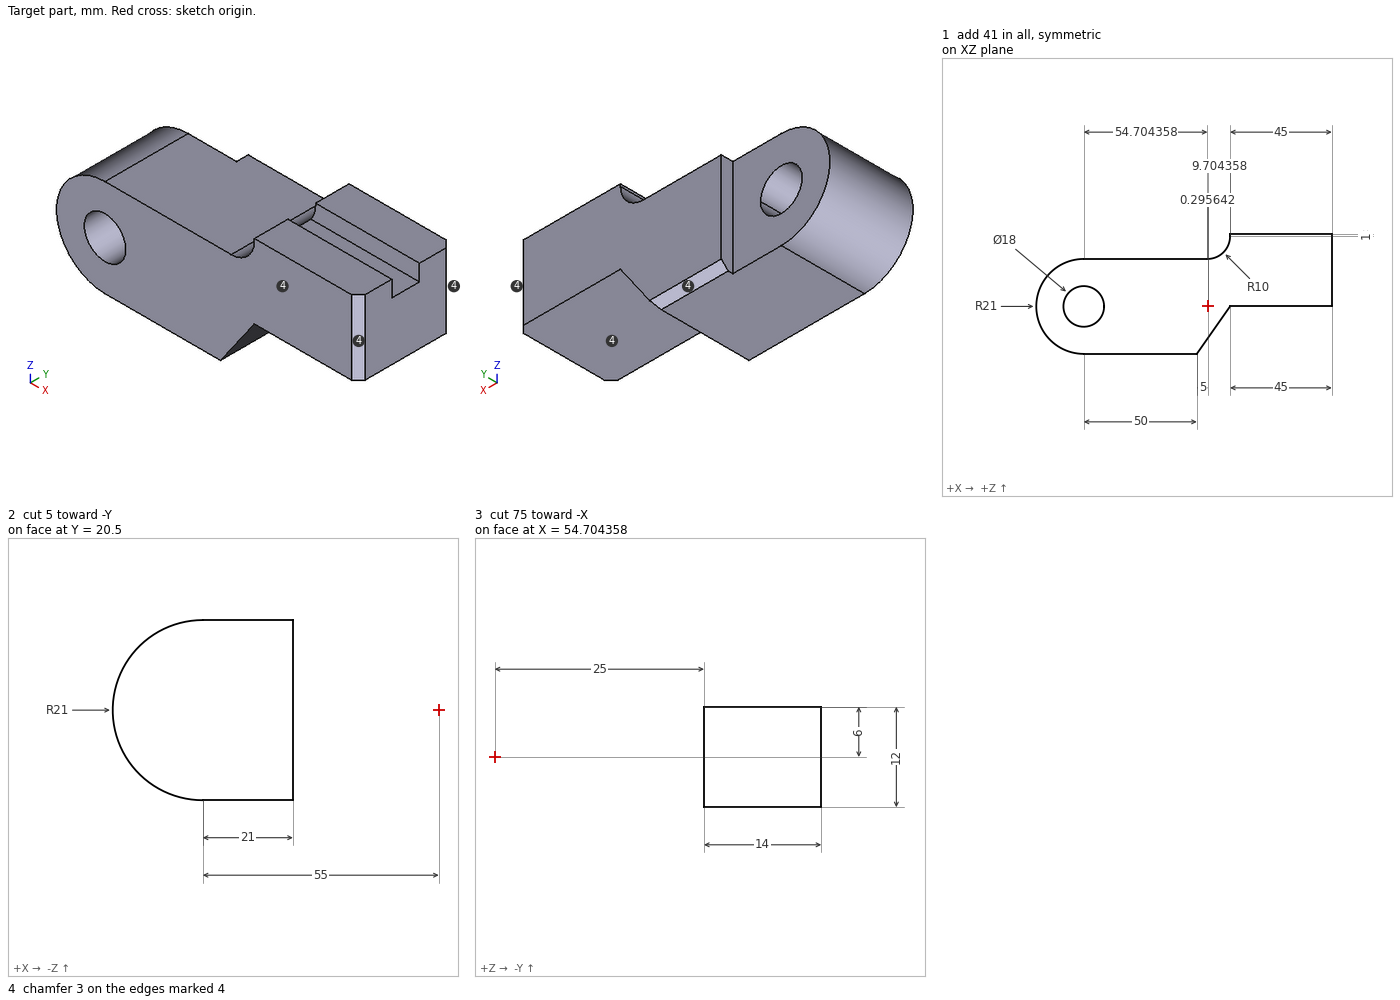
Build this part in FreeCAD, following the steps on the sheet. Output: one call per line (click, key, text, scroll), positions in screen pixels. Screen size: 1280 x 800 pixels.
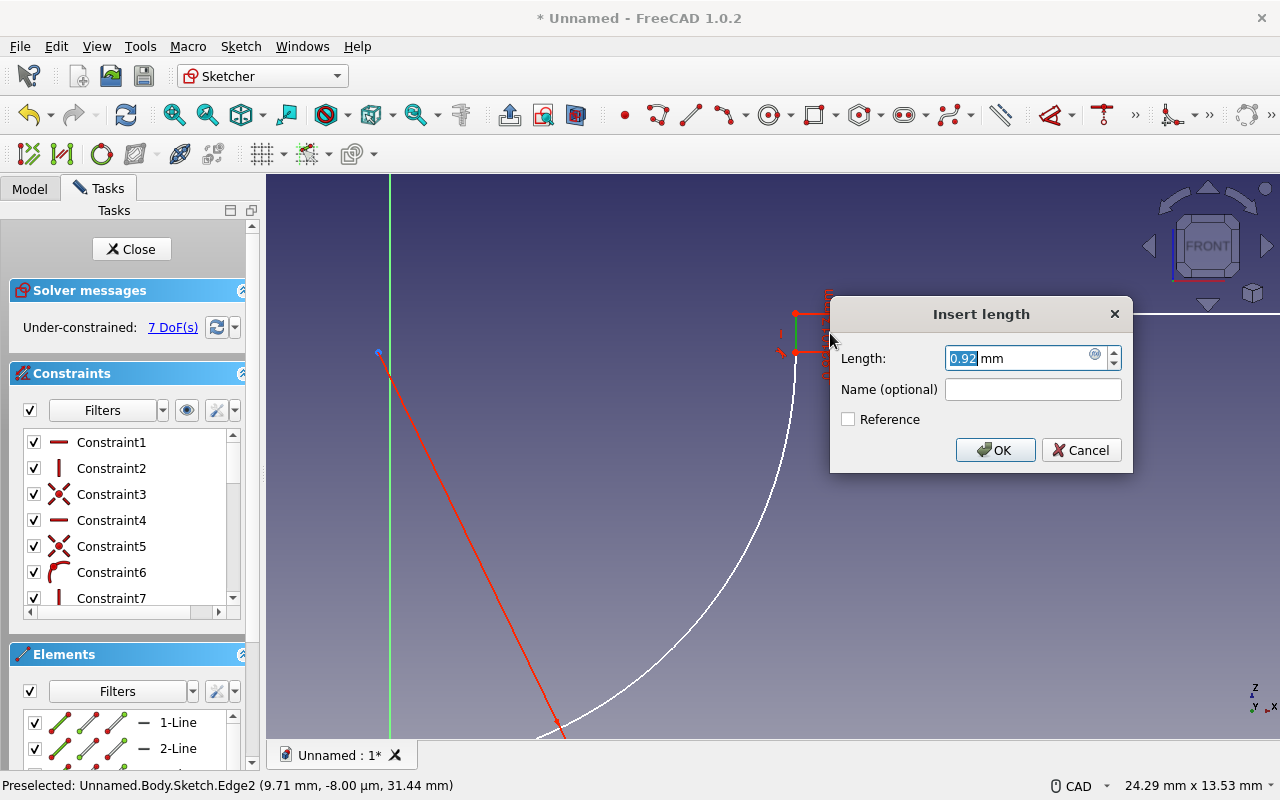
text(1)
key(Return)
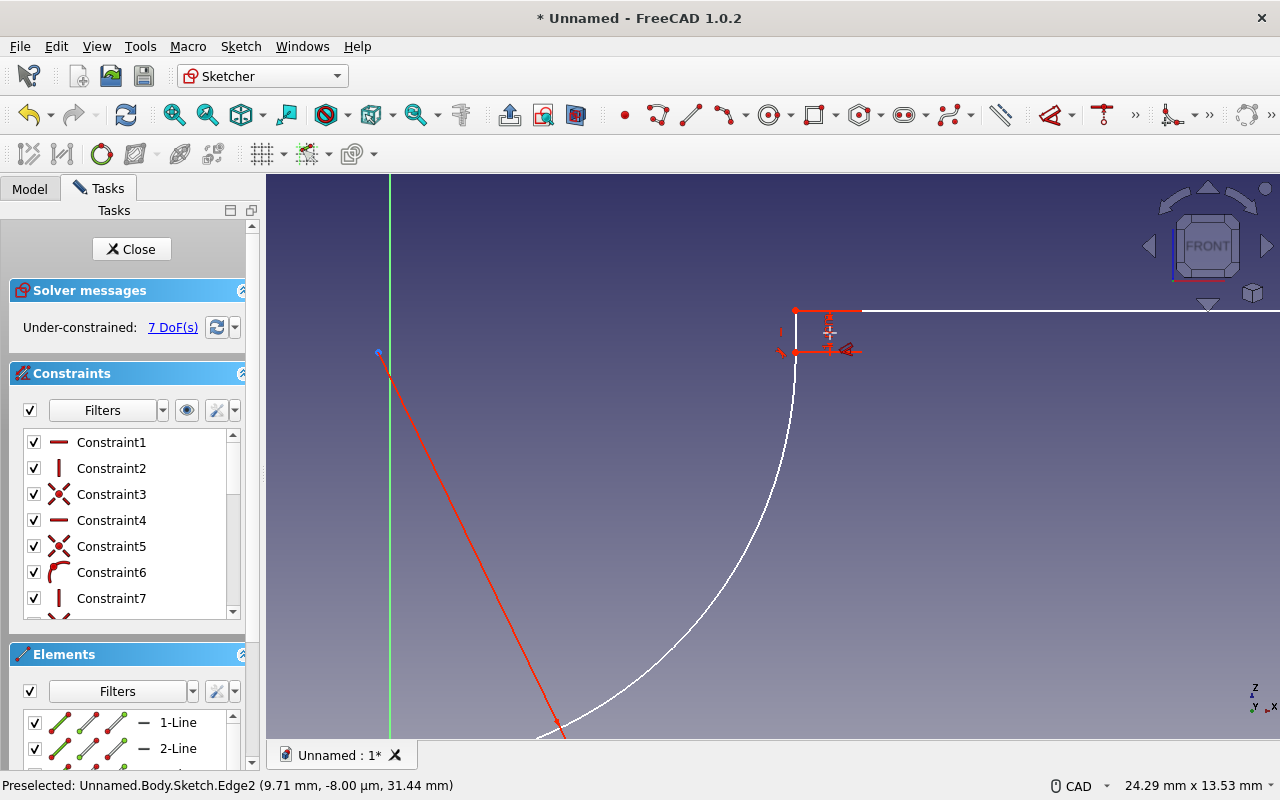
scroll(799, 337, down, 11)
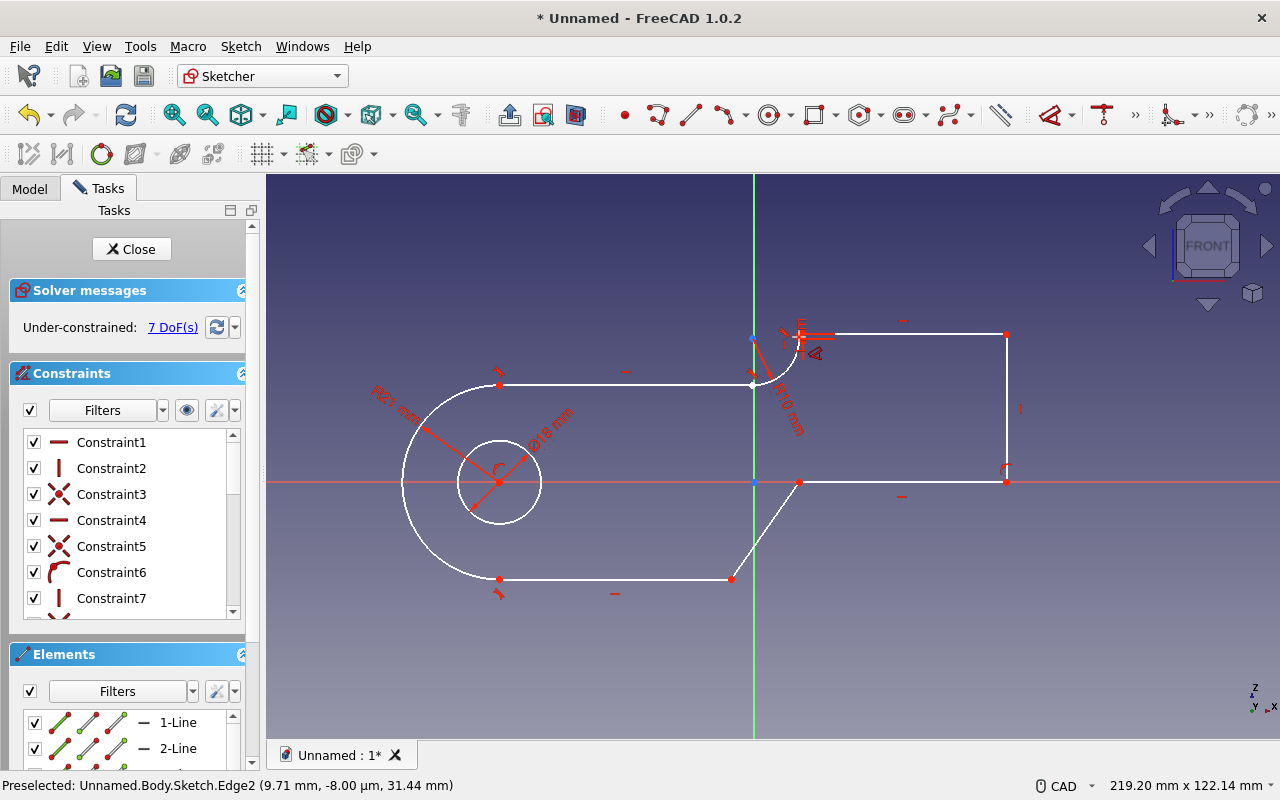
click(861, 334)
click(903, 300)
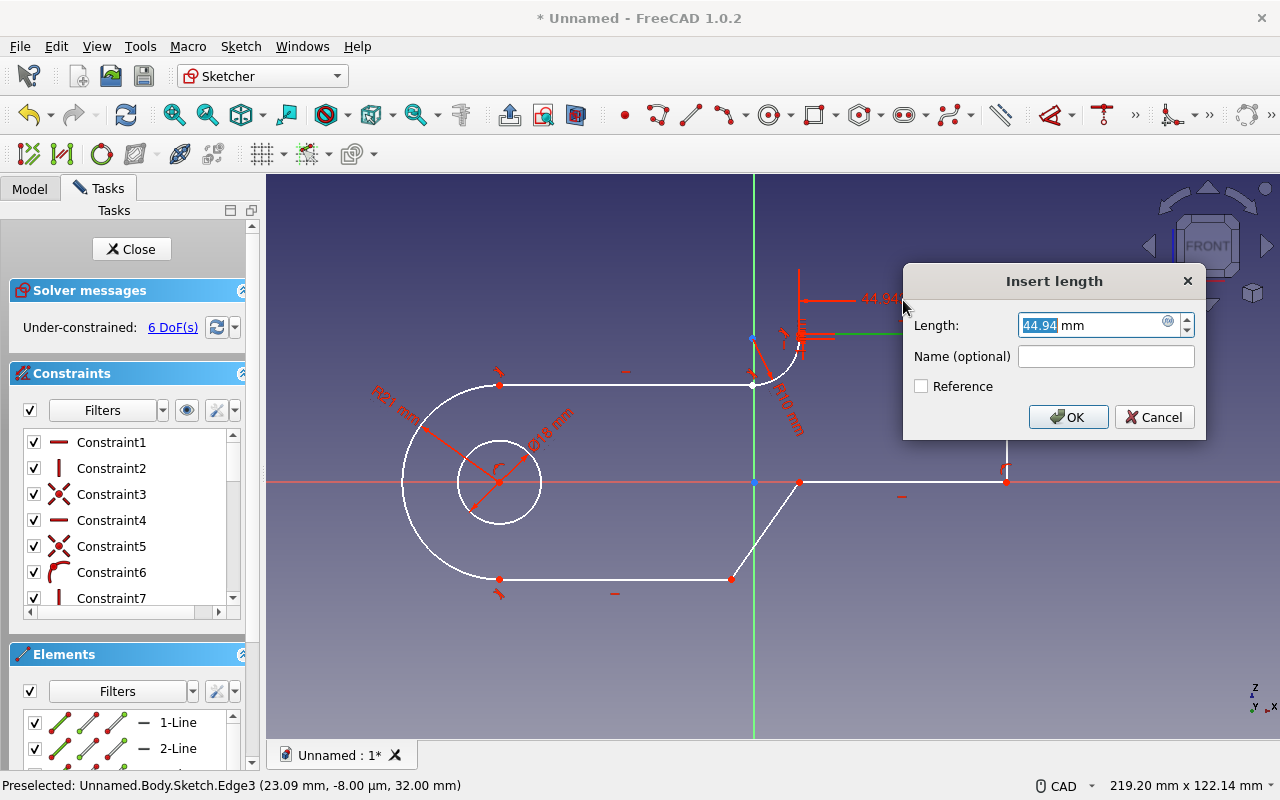
text(45)
key(Return)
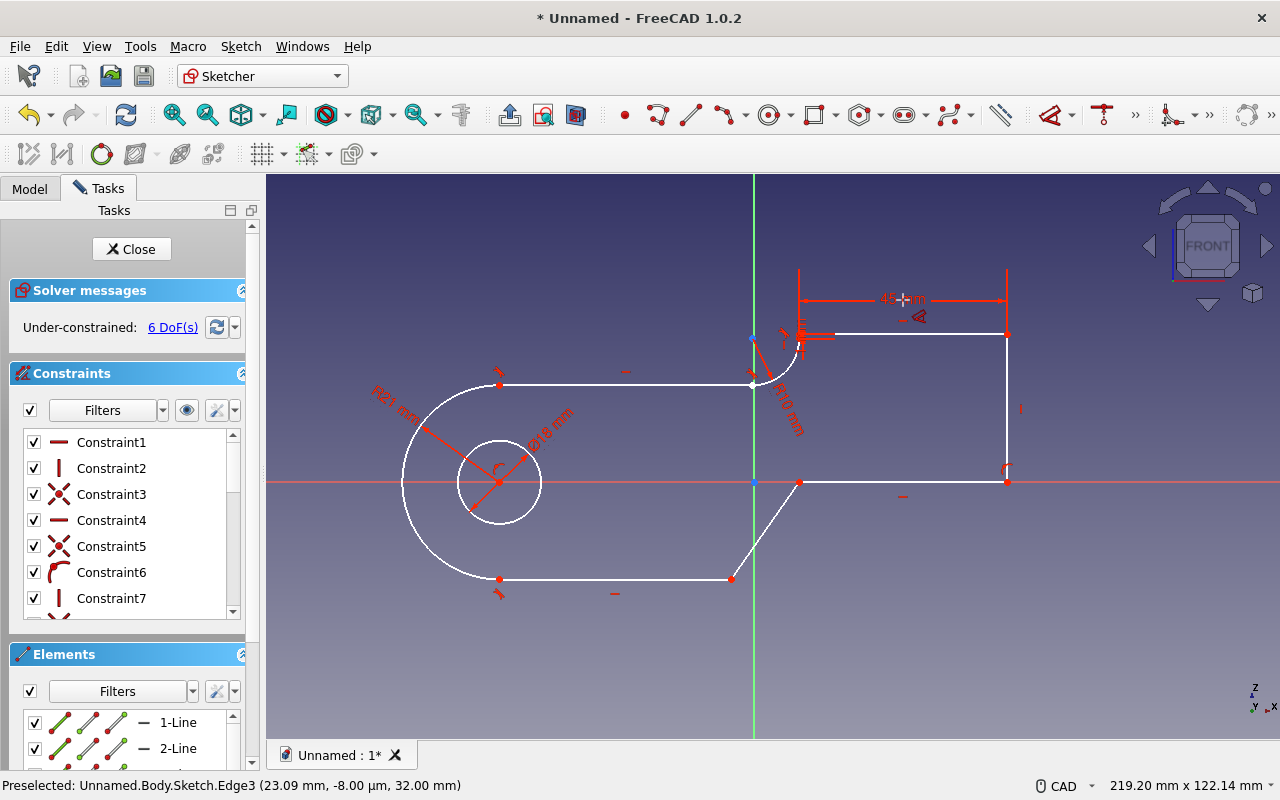
click(945, 482)
click(903, 516)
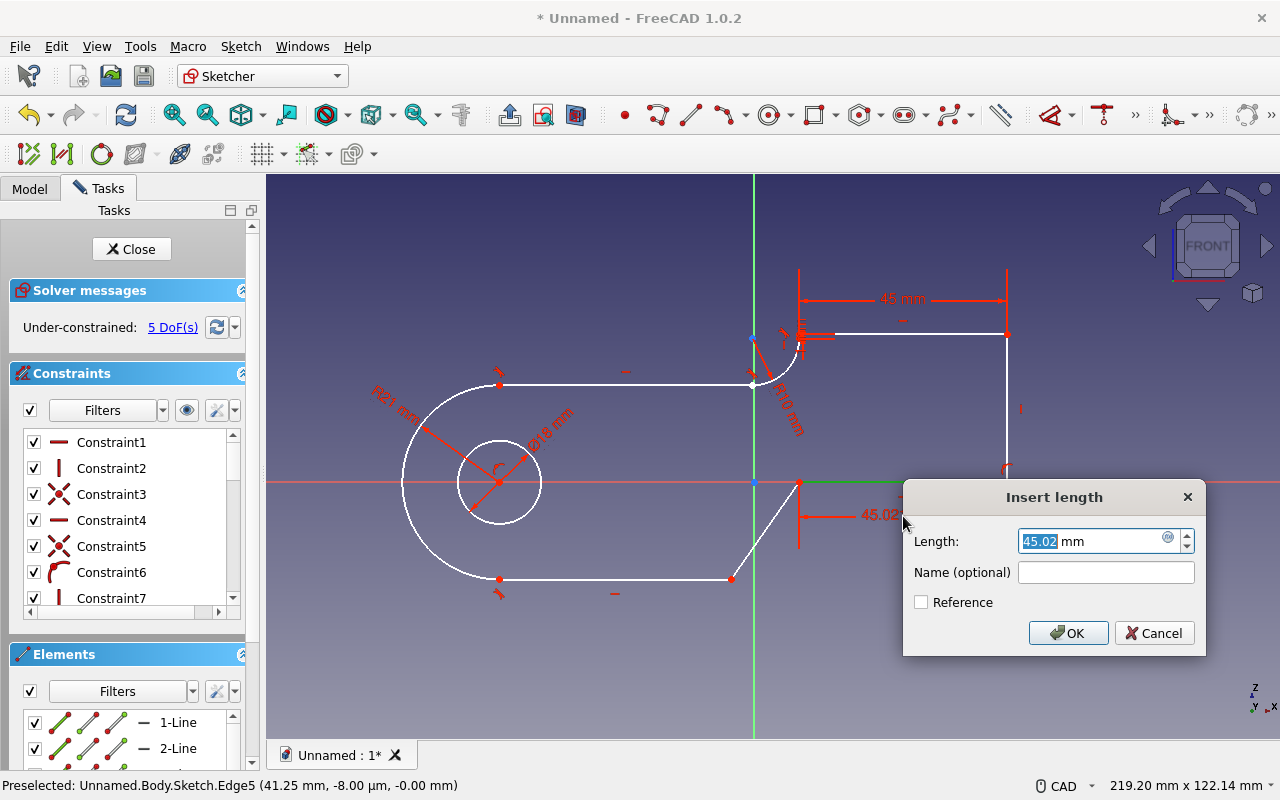
text(45)
key(Return)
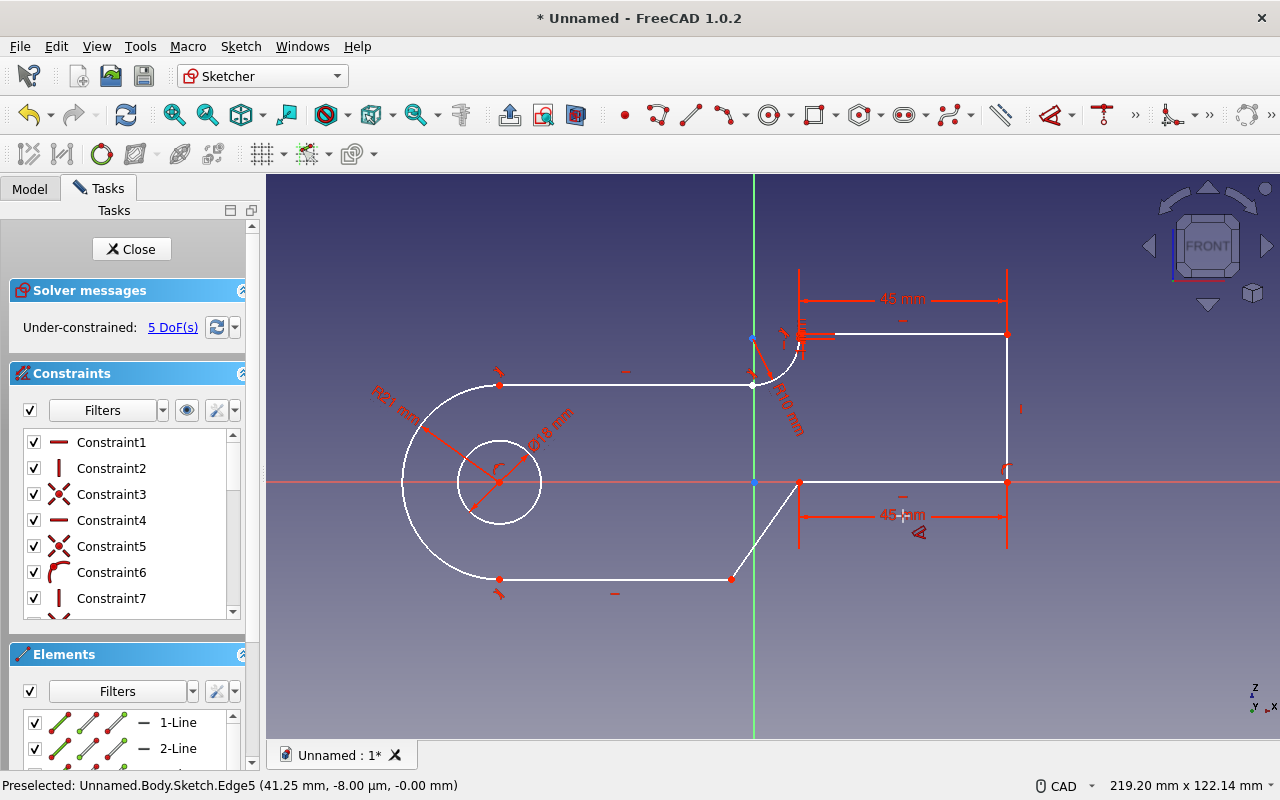
click(662, 580)
click(615, 614)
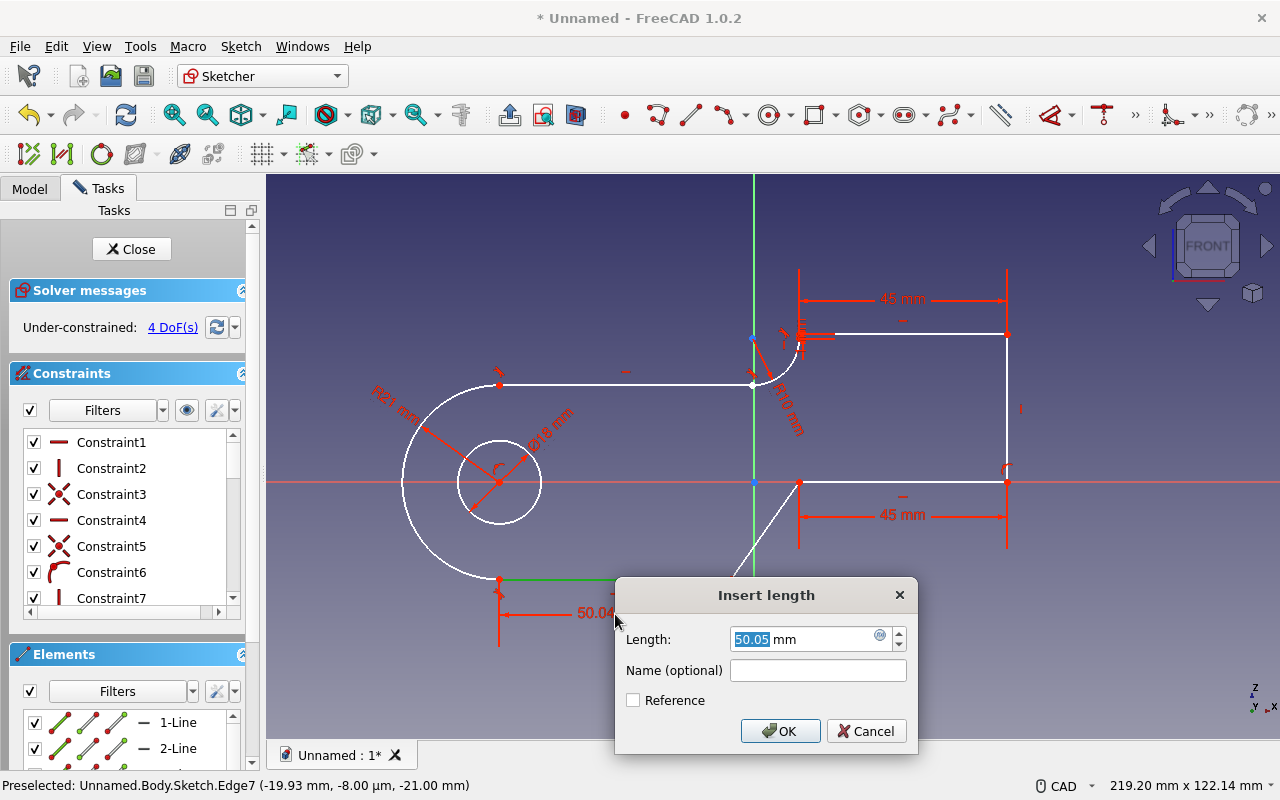
text(50)
key(Return)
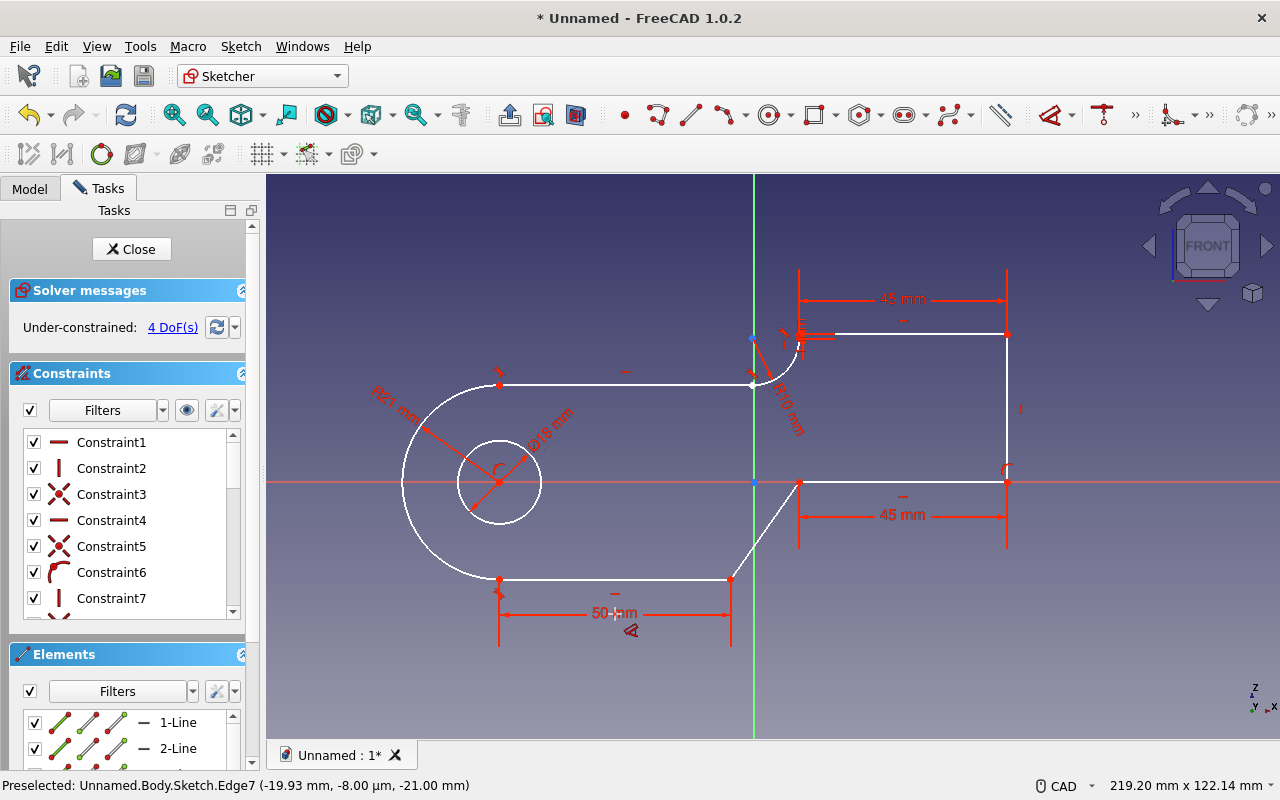
scroll(731, 580, up, 3)